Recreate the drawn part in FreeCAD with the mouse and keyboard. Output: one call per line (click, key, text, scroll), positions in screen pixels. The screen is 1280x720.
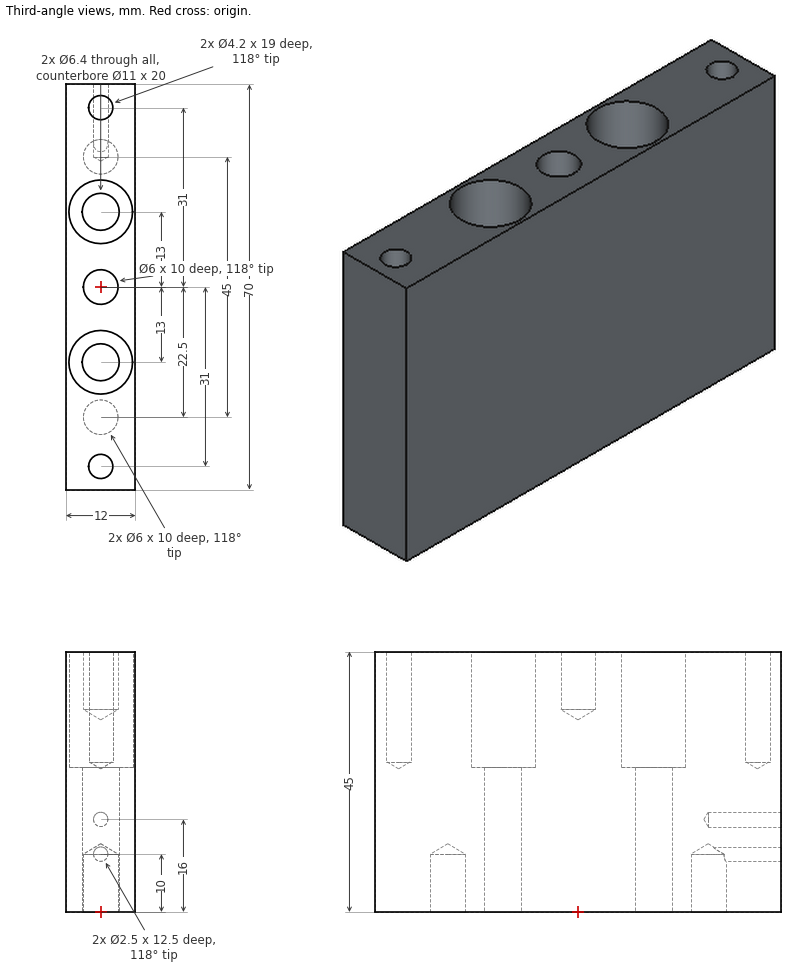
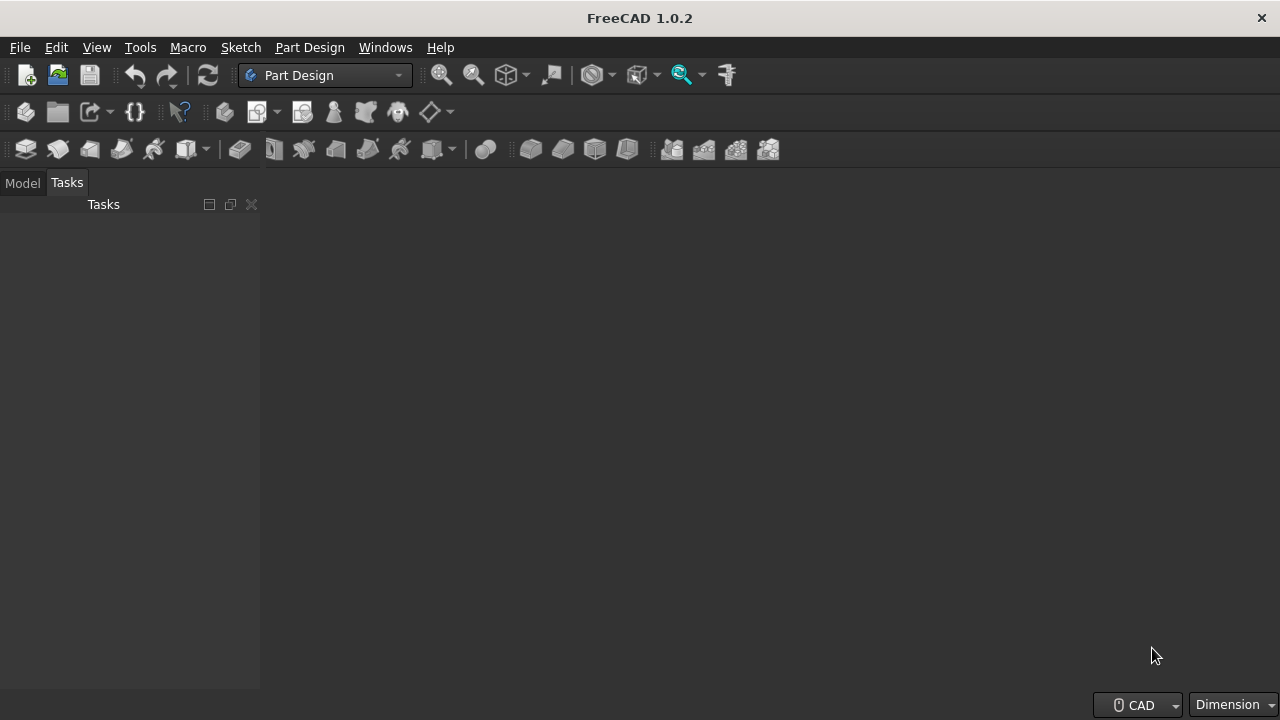
click(26, 76)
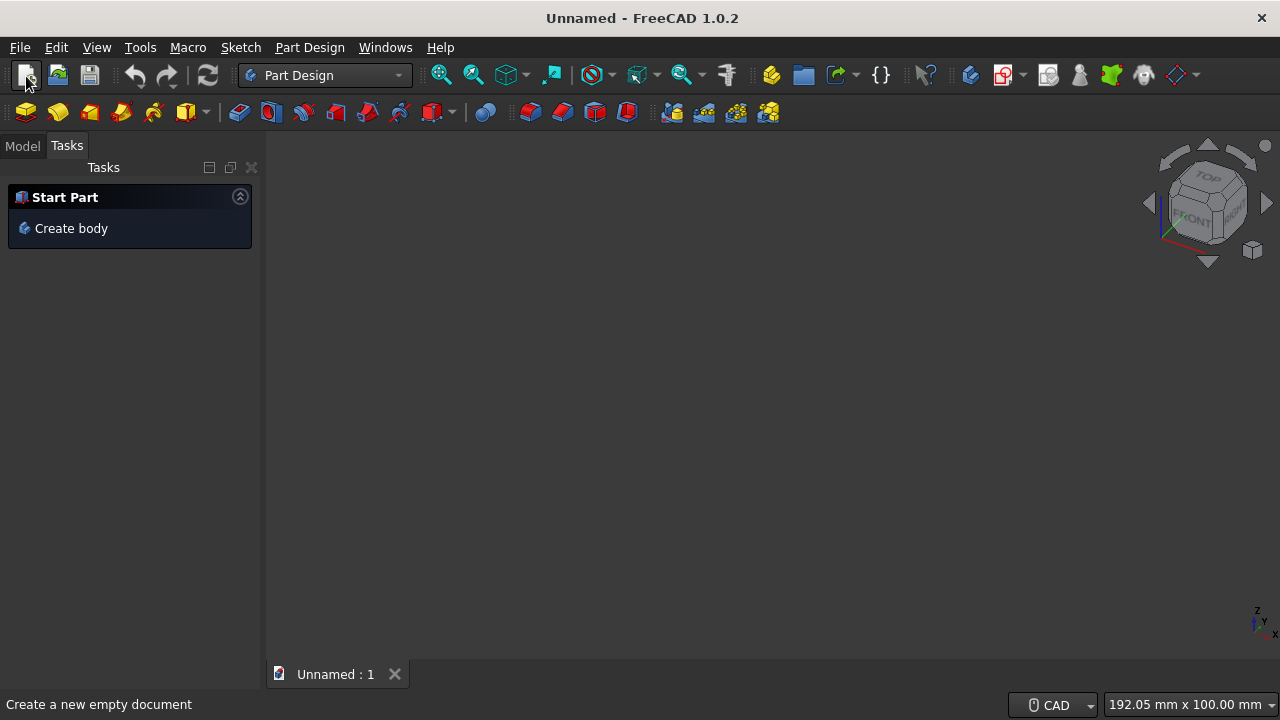
click(1004, 76)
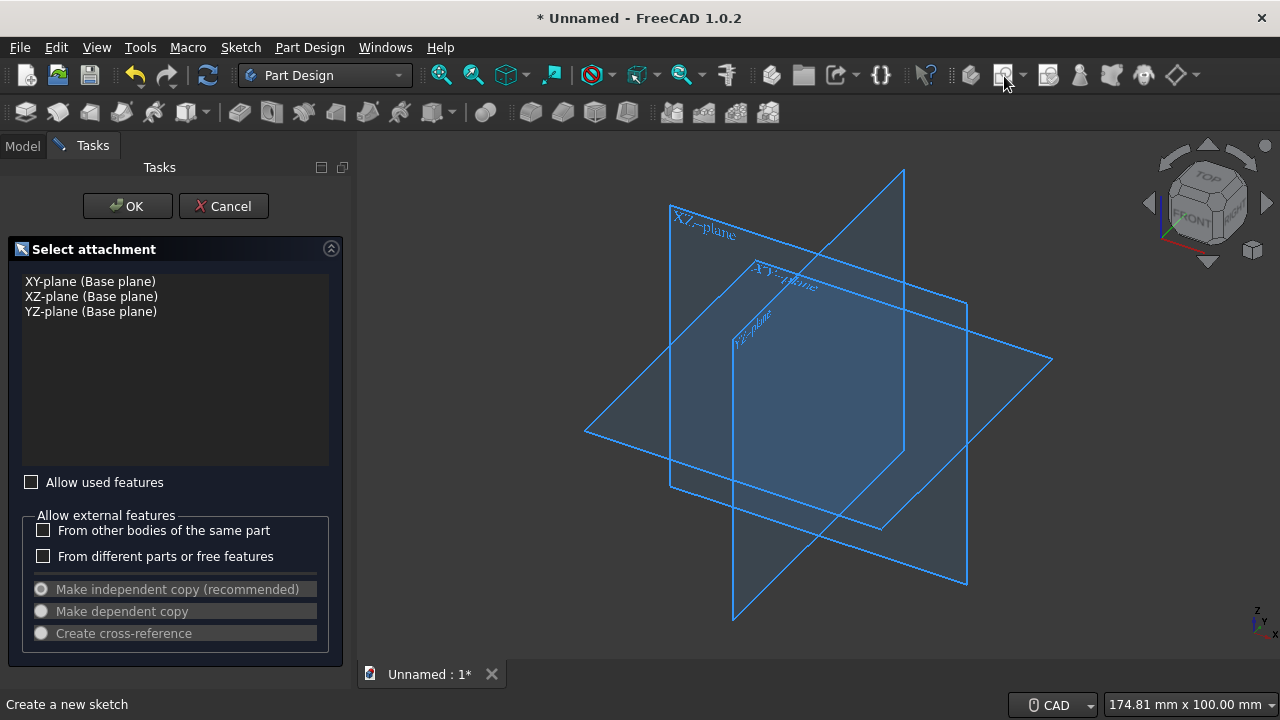
click(82, 282)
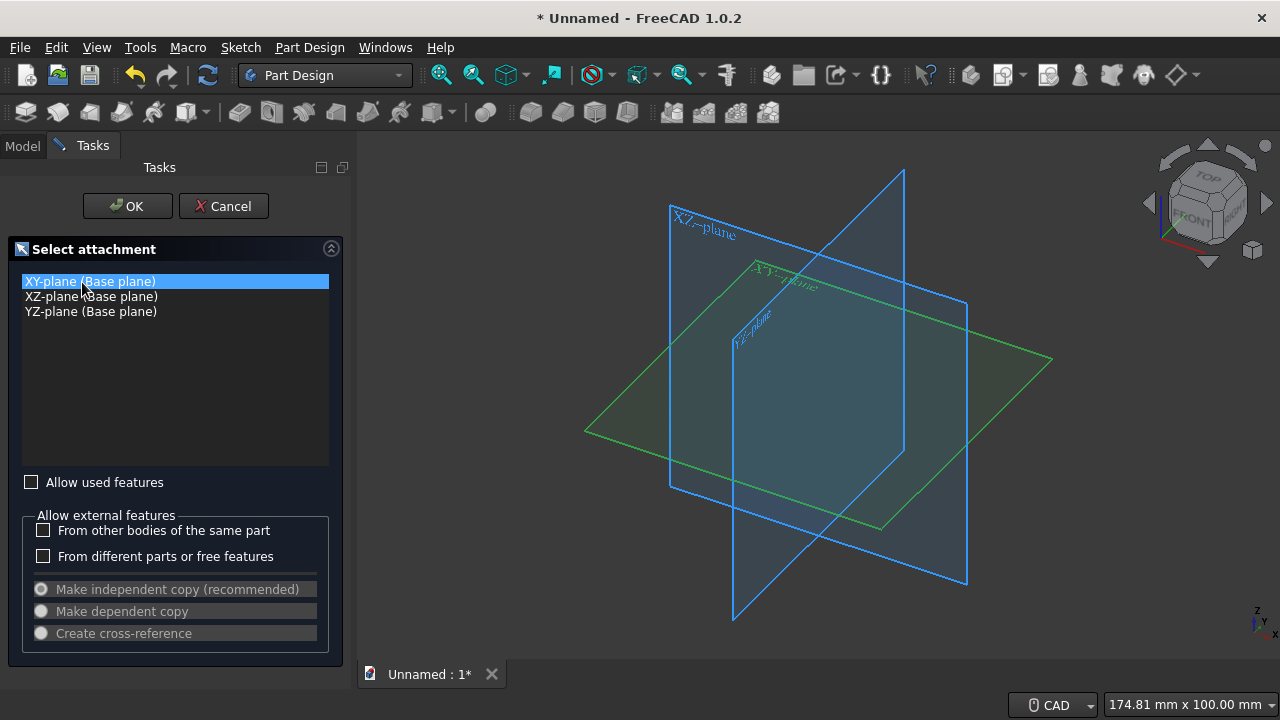
click(128, 206)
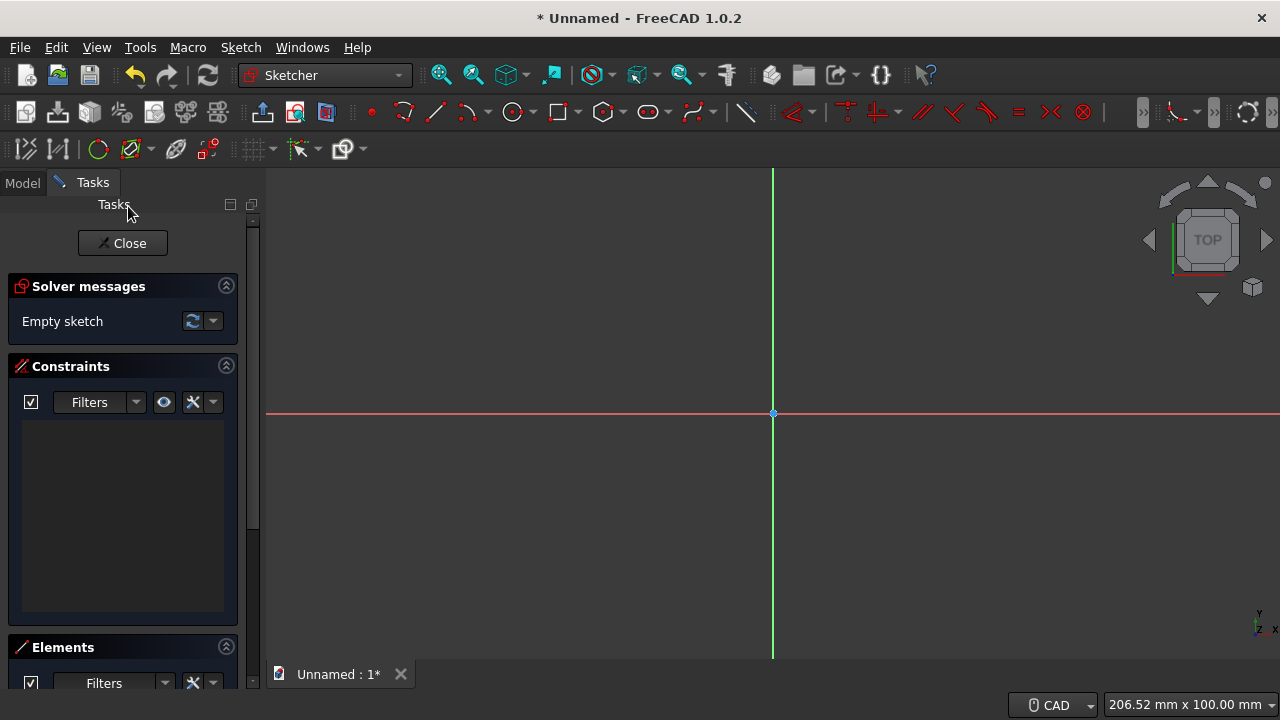
key(g)
key(v)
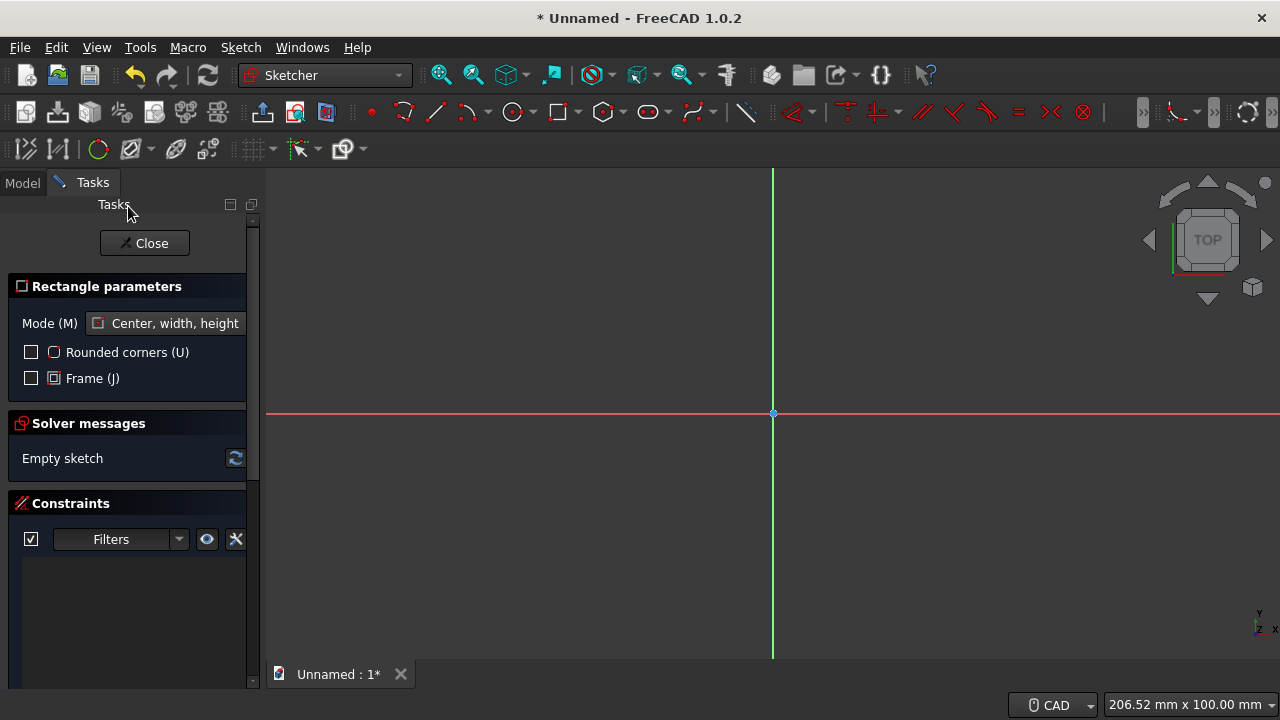
click(773, 414)
move(802, 242)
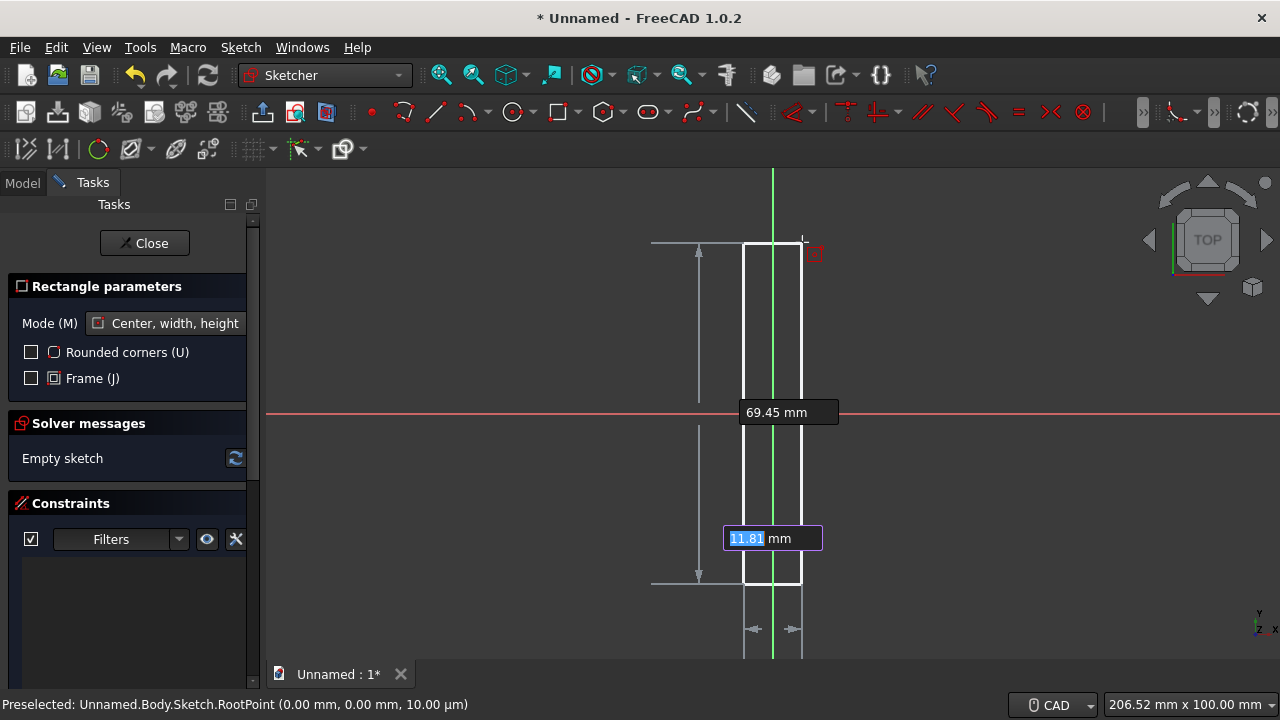
text(12)
key(Tab)
text(70)
key(Return)
key(Escape)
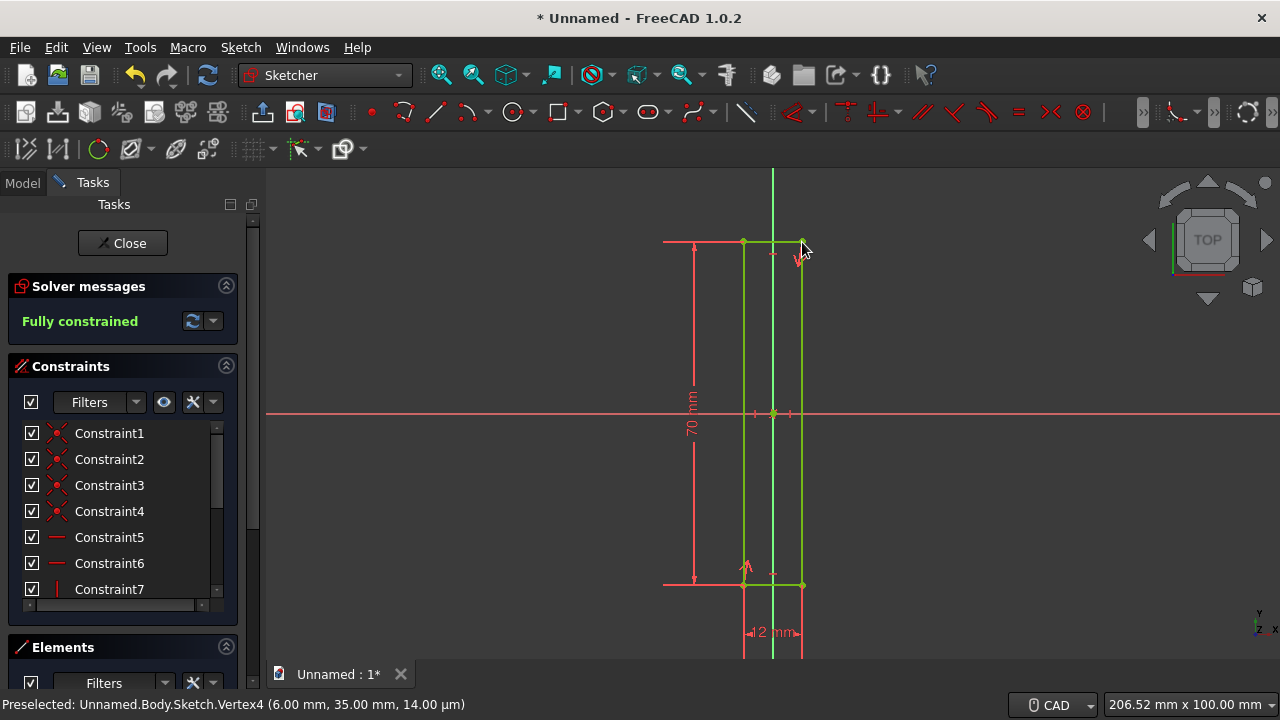
click(123, 243)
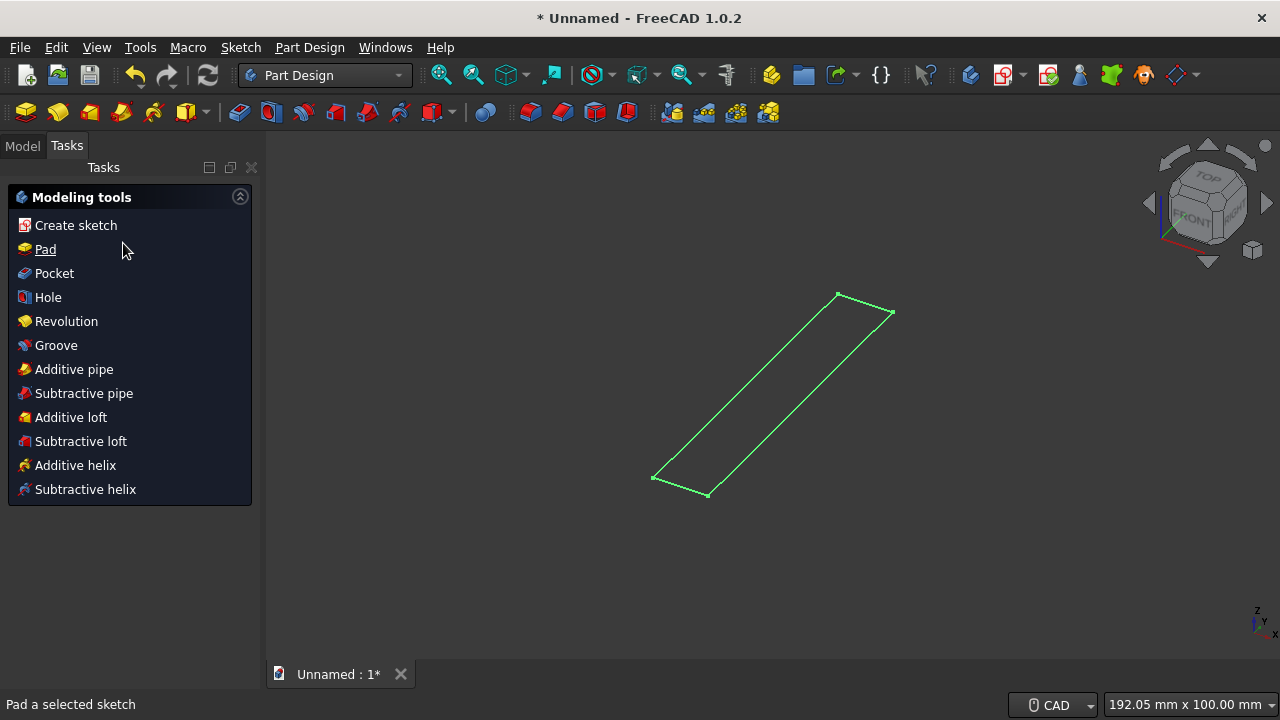
click(26, 112)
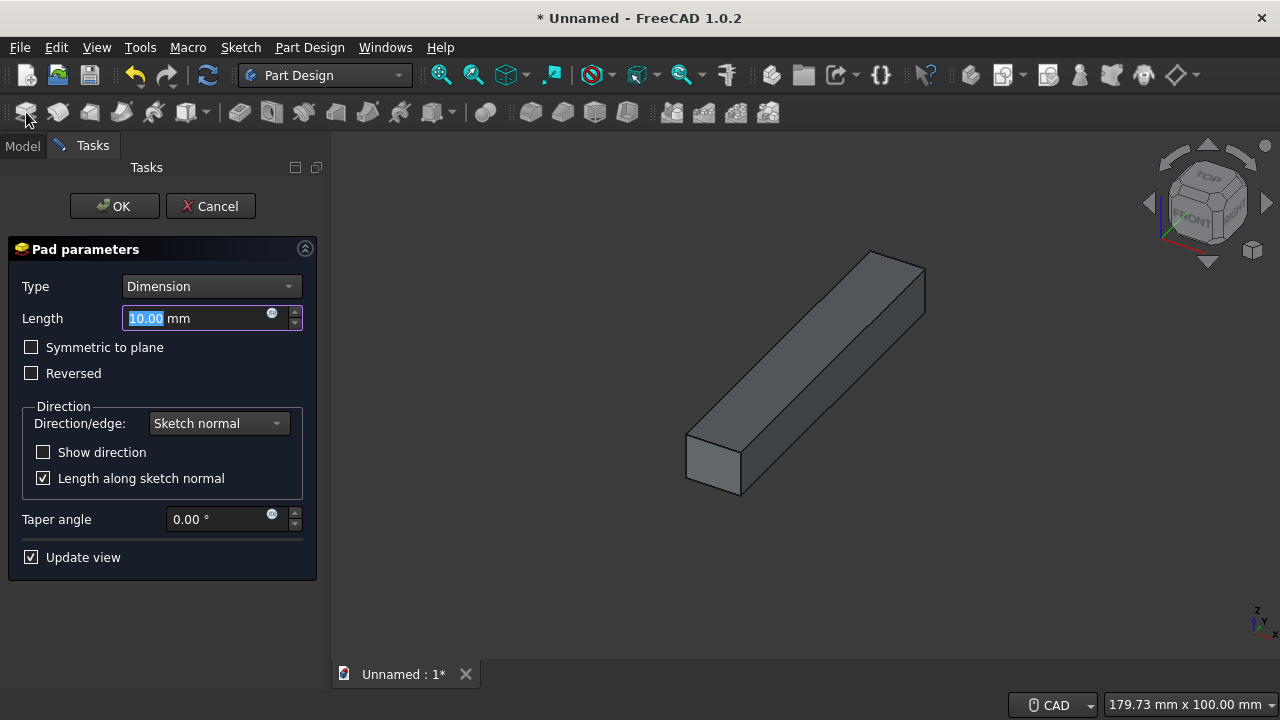
text(45)
key(Tab)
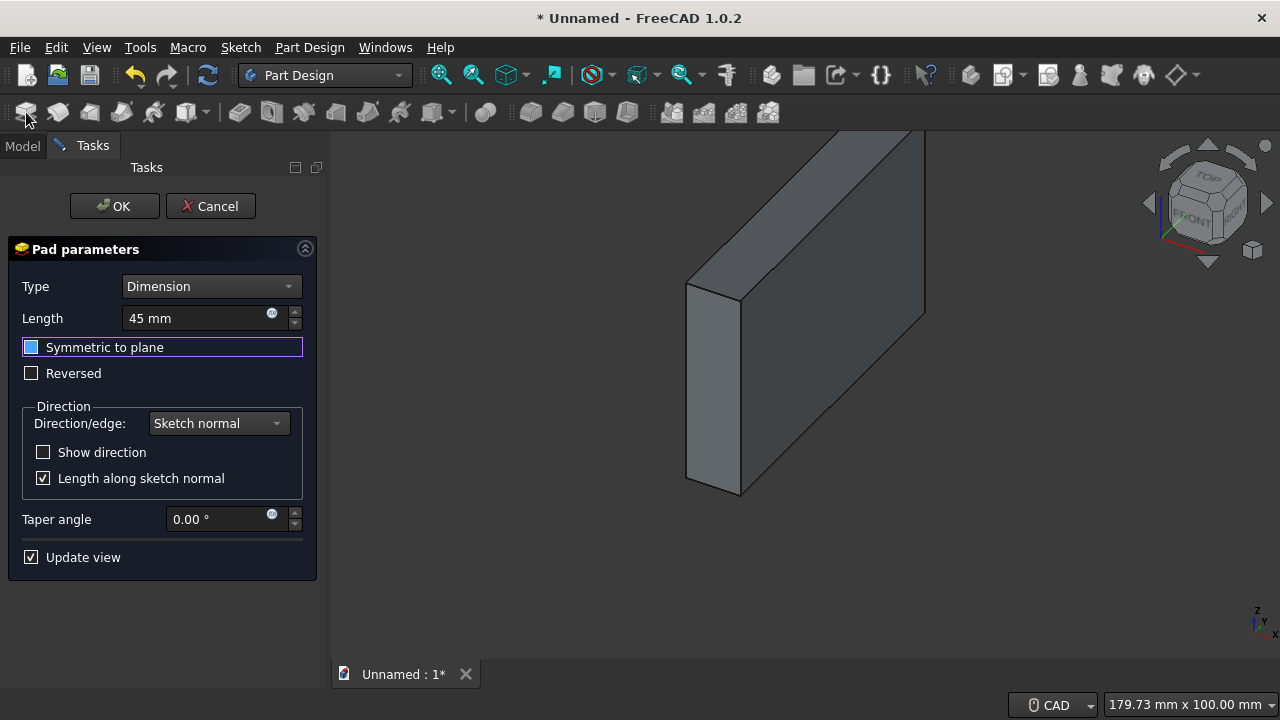
click(115, 206)